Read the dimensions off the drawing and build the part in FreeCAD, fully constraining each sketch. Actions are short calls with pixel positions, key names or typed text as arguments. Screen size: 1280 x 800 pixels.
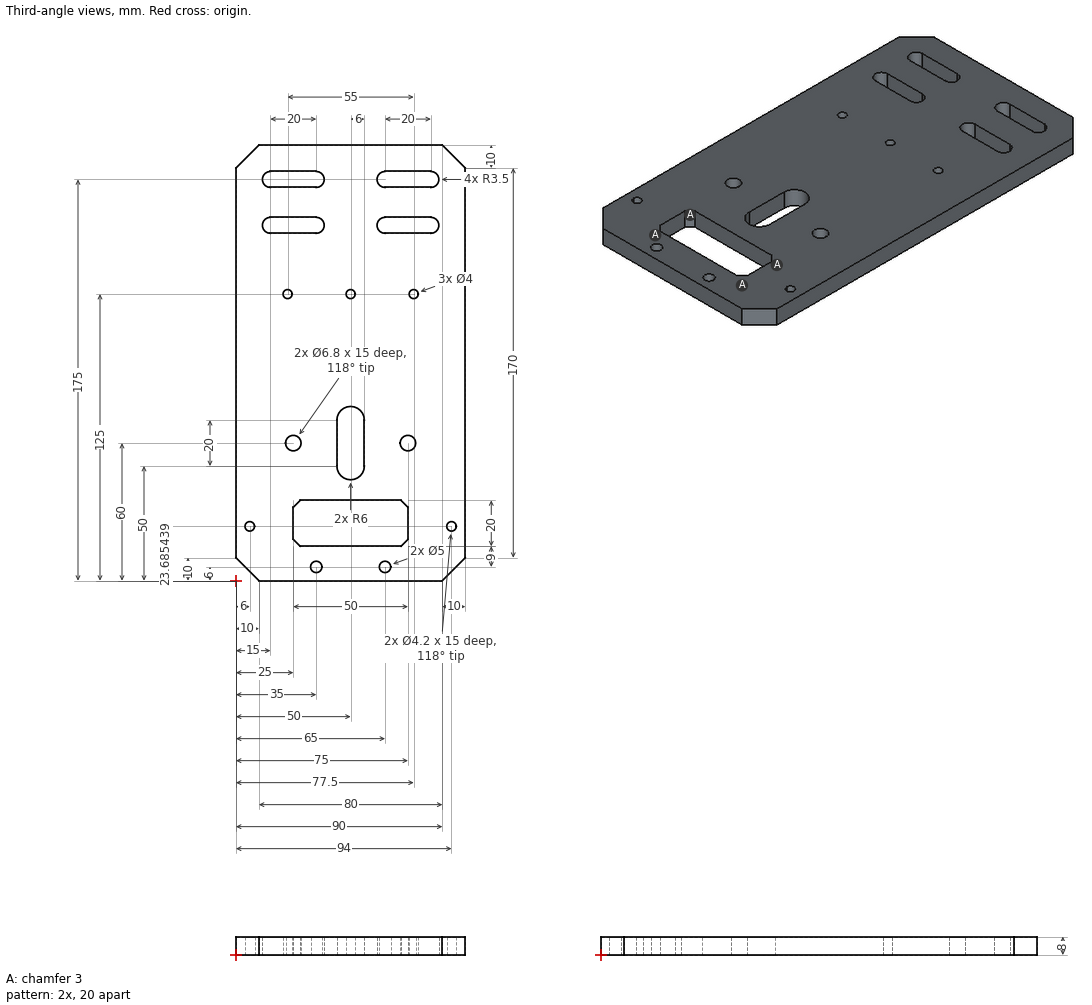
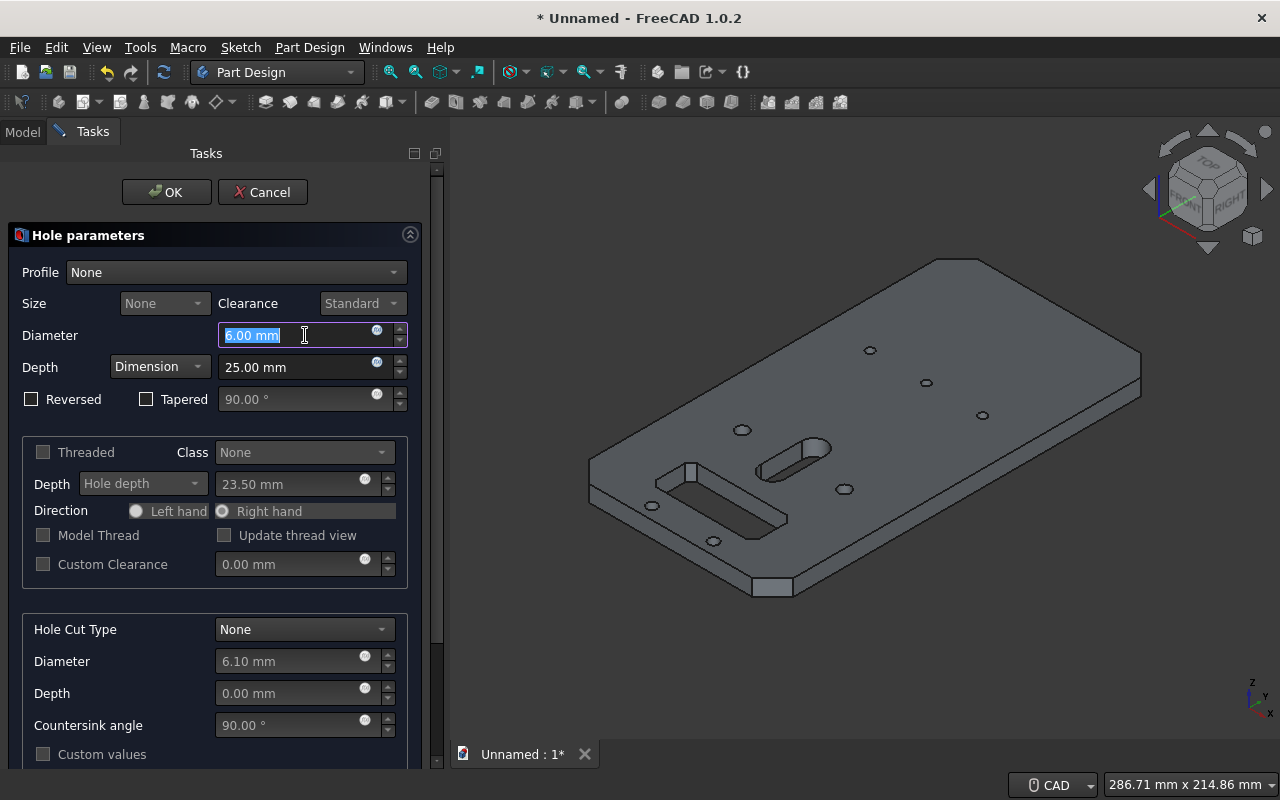
text(6.8)
key(Tab)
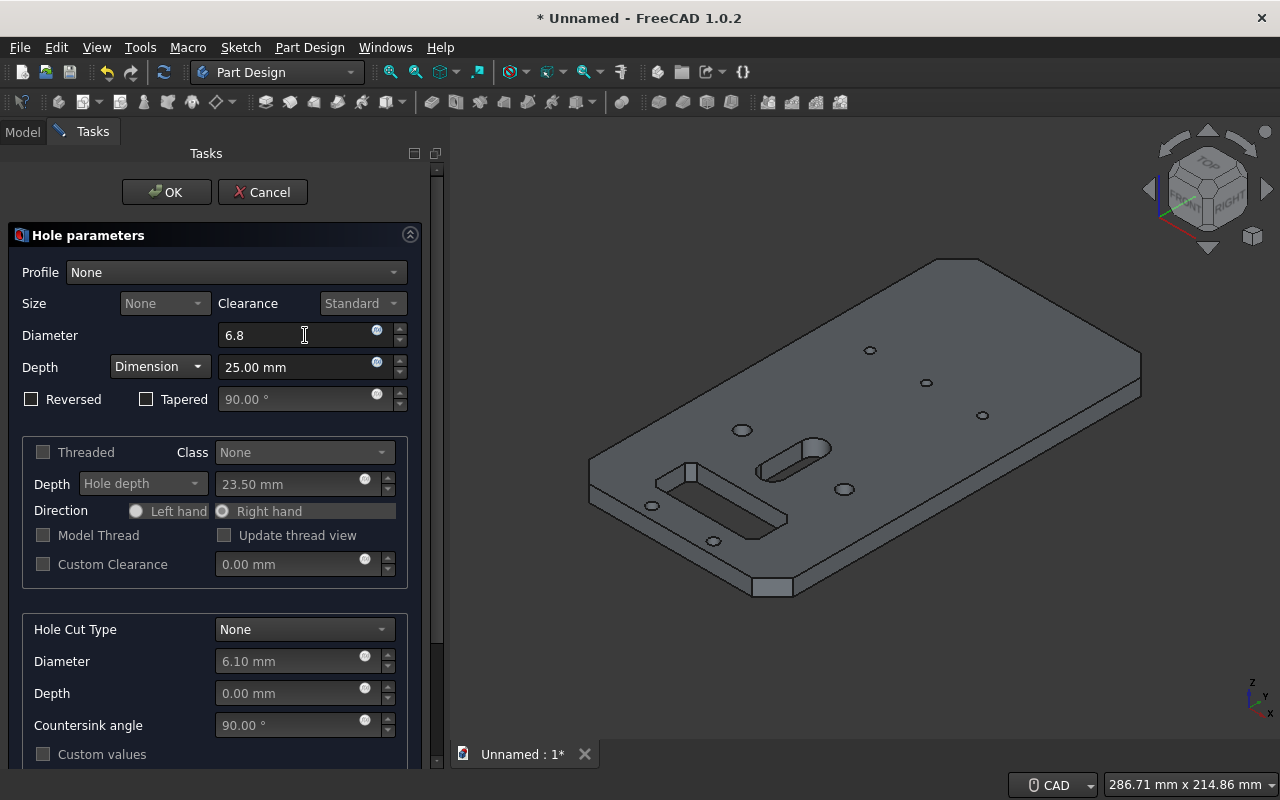
triple_click(305, 367)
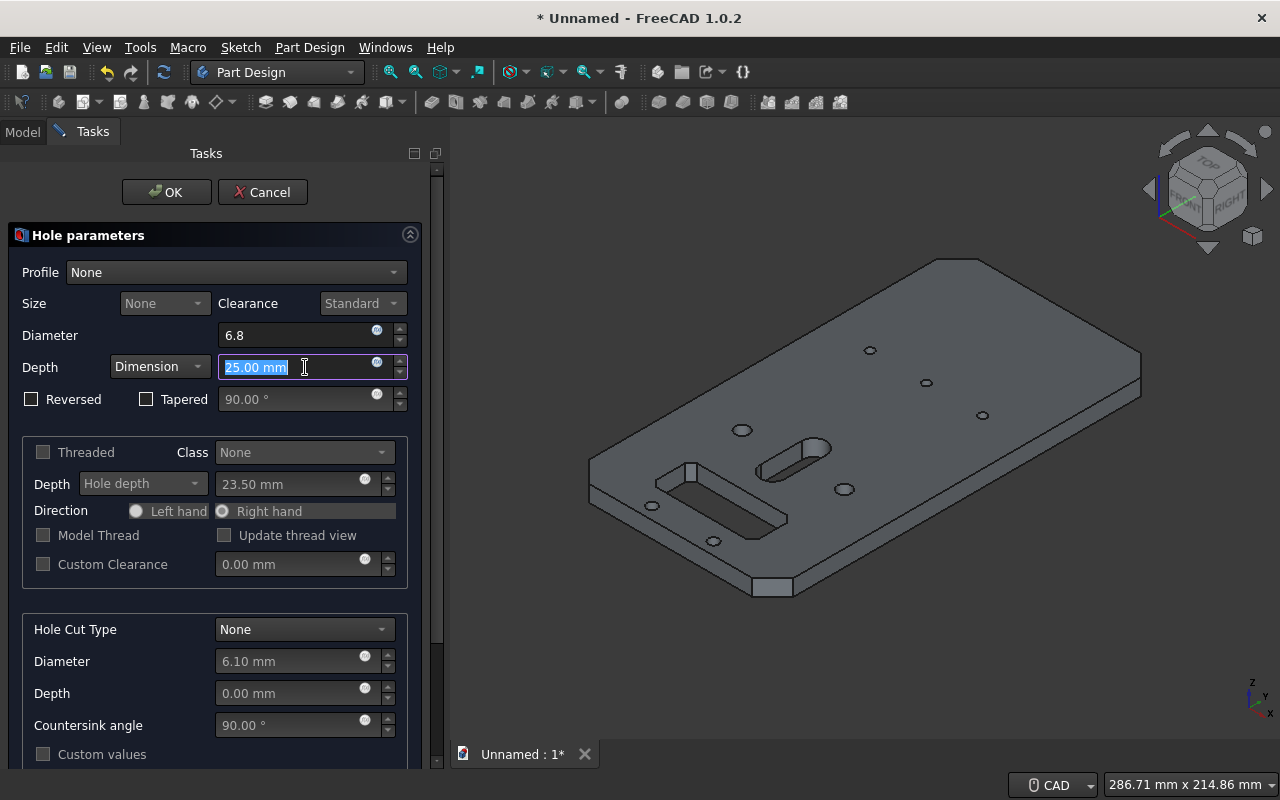
text(15)
key(Tab)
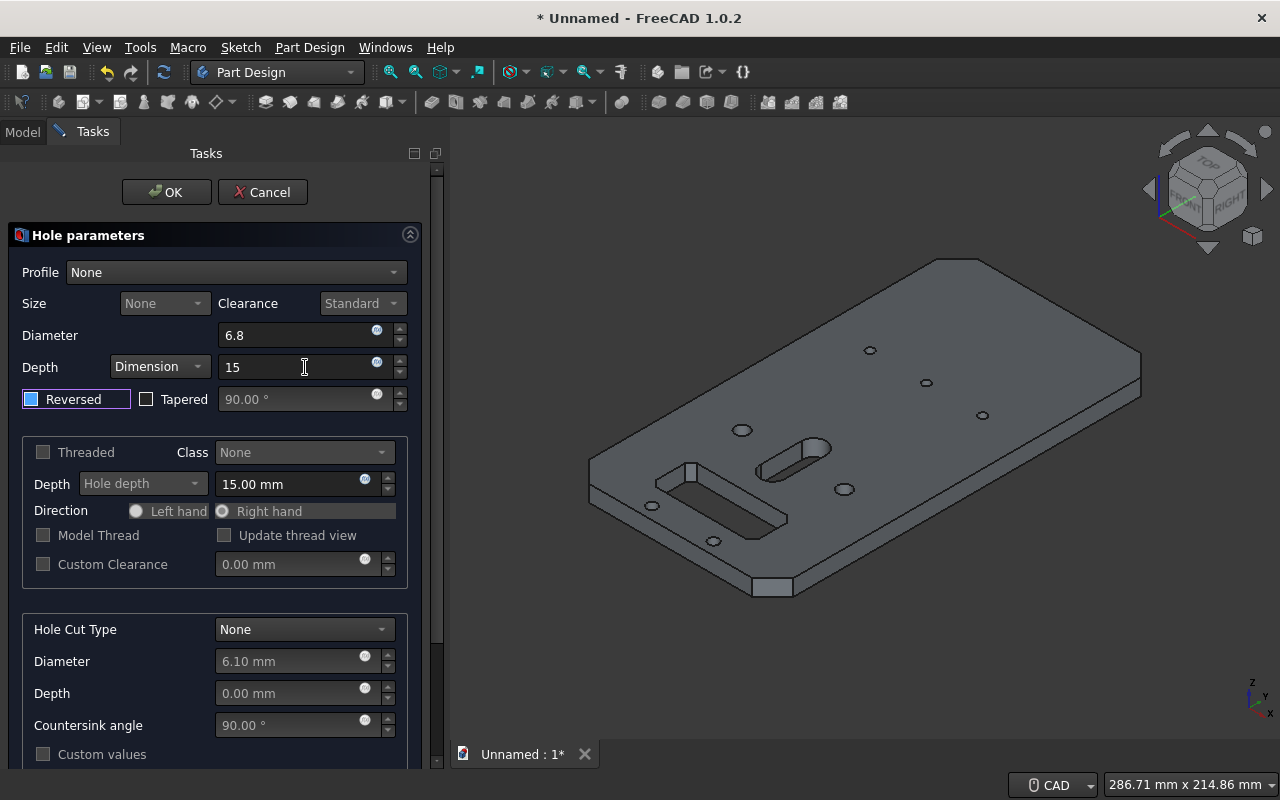
click(167, 192)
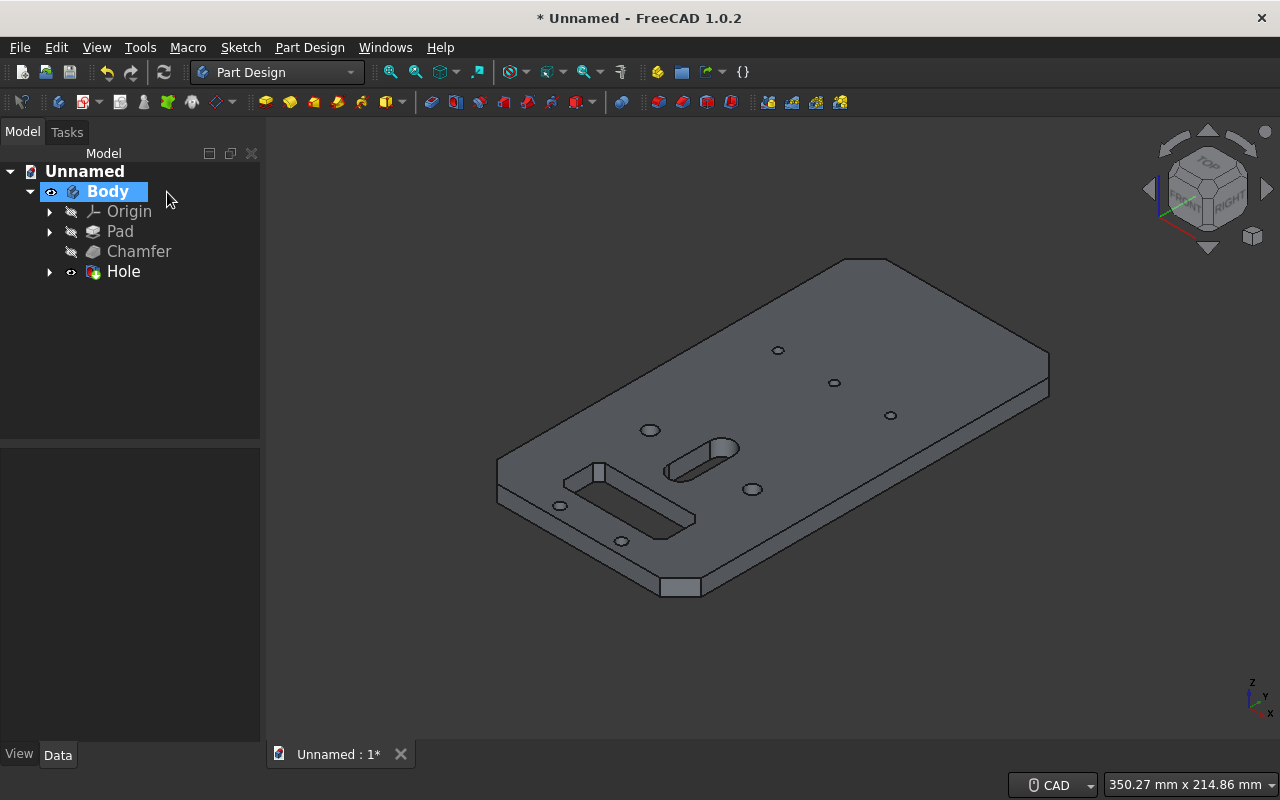
key(5)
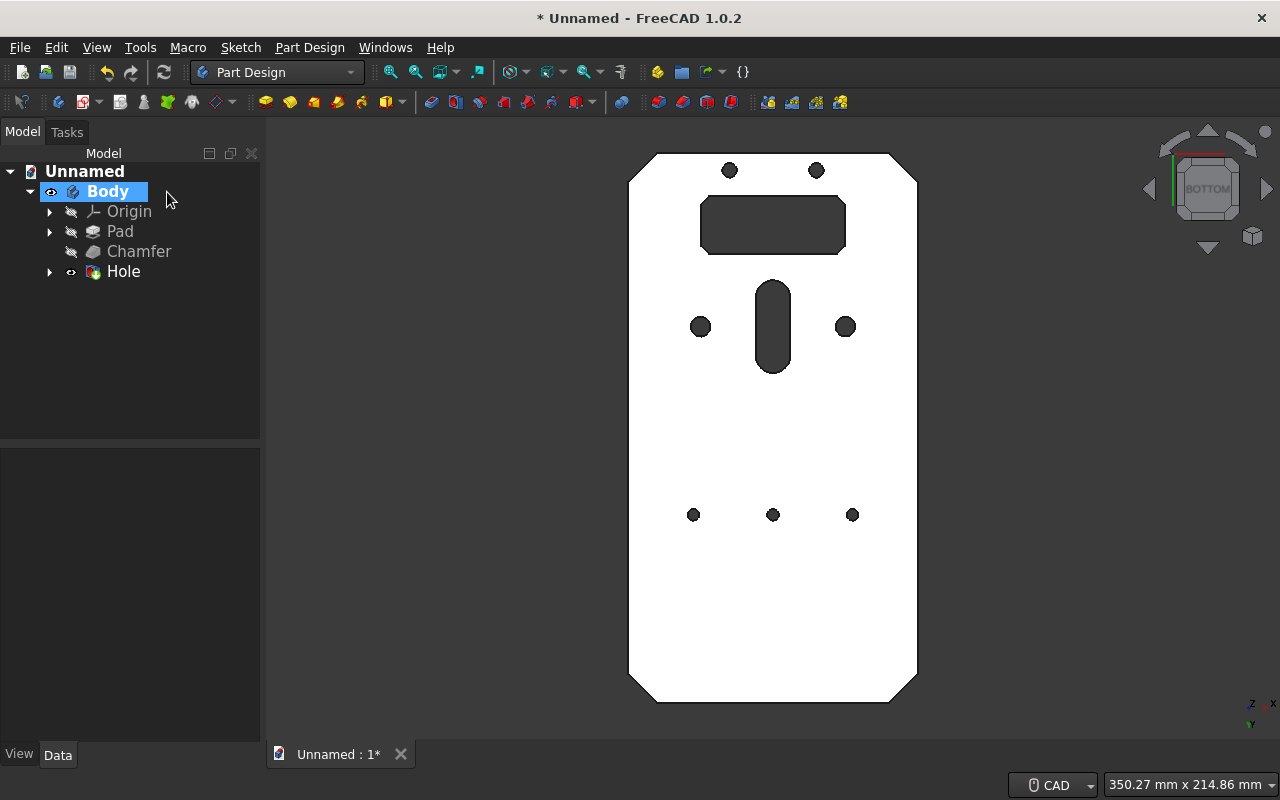
click(814, 584)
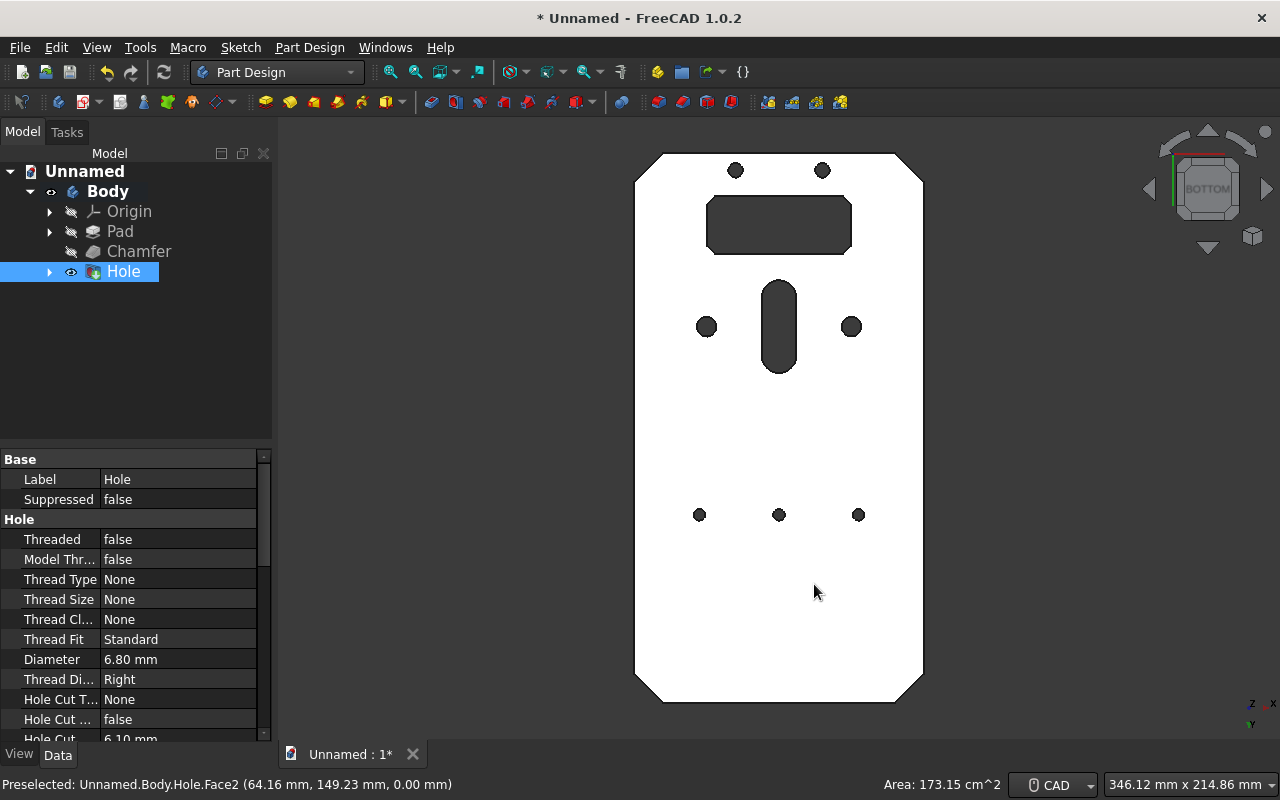
click(84, 102)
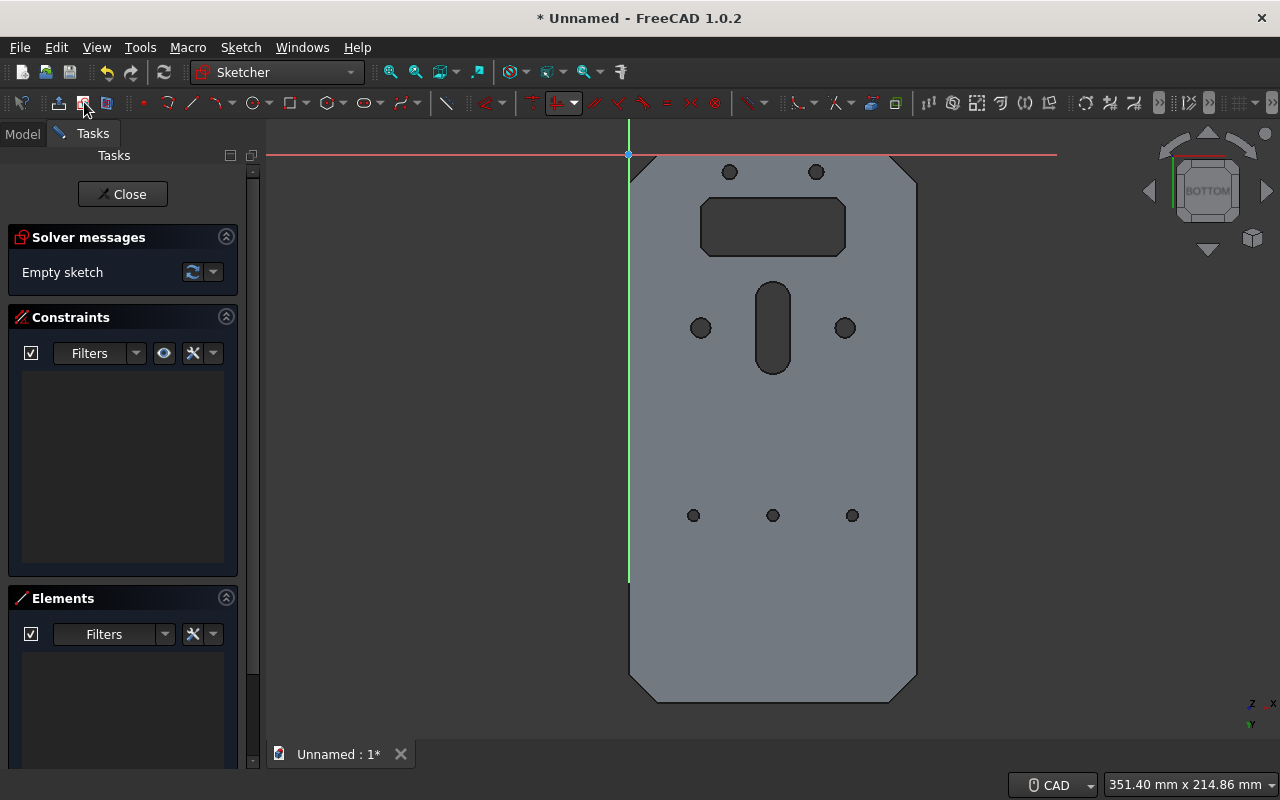
scroll(704, 429, down, 5)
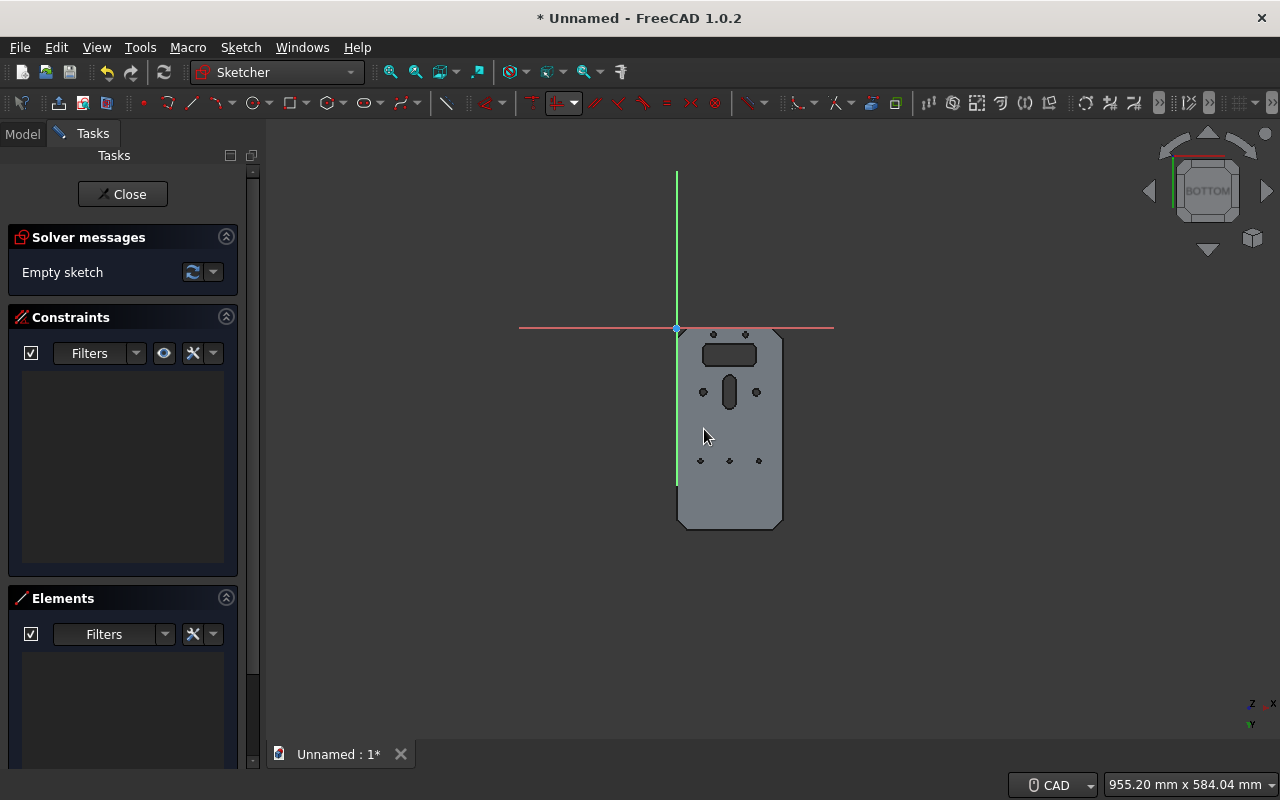
scroll(732, 325, up, 9)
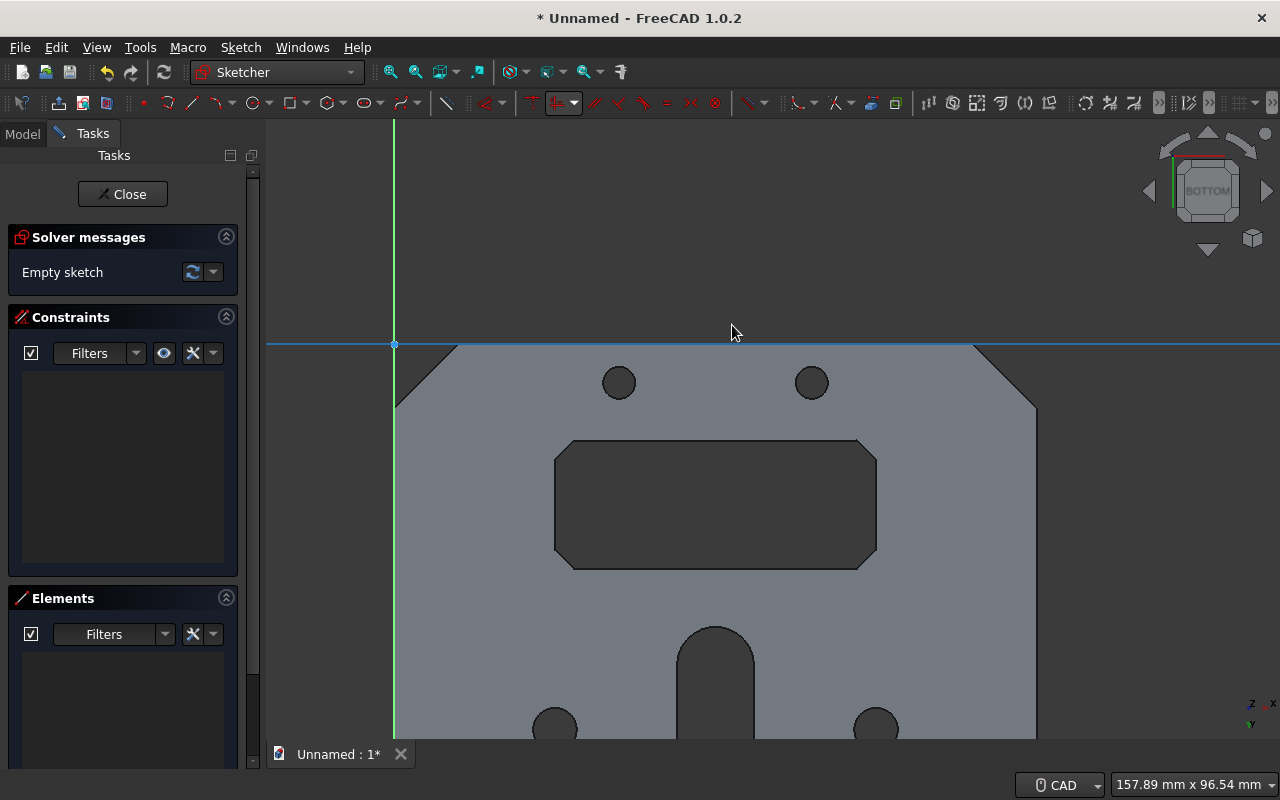
key(g)
key(c)